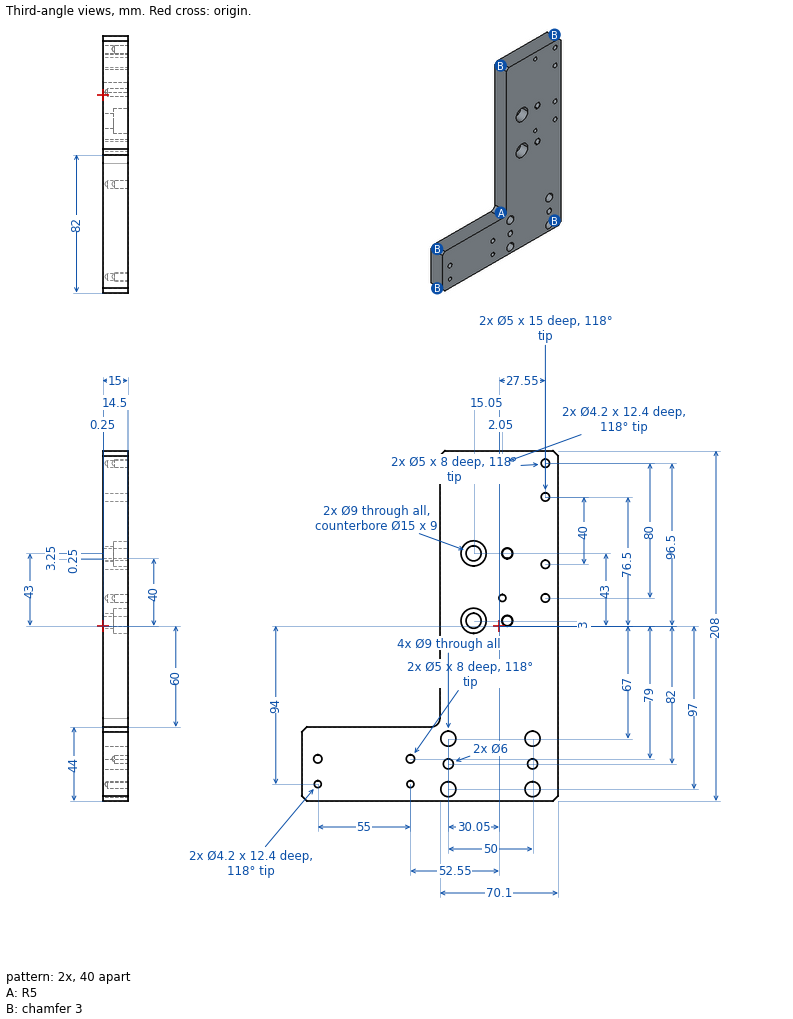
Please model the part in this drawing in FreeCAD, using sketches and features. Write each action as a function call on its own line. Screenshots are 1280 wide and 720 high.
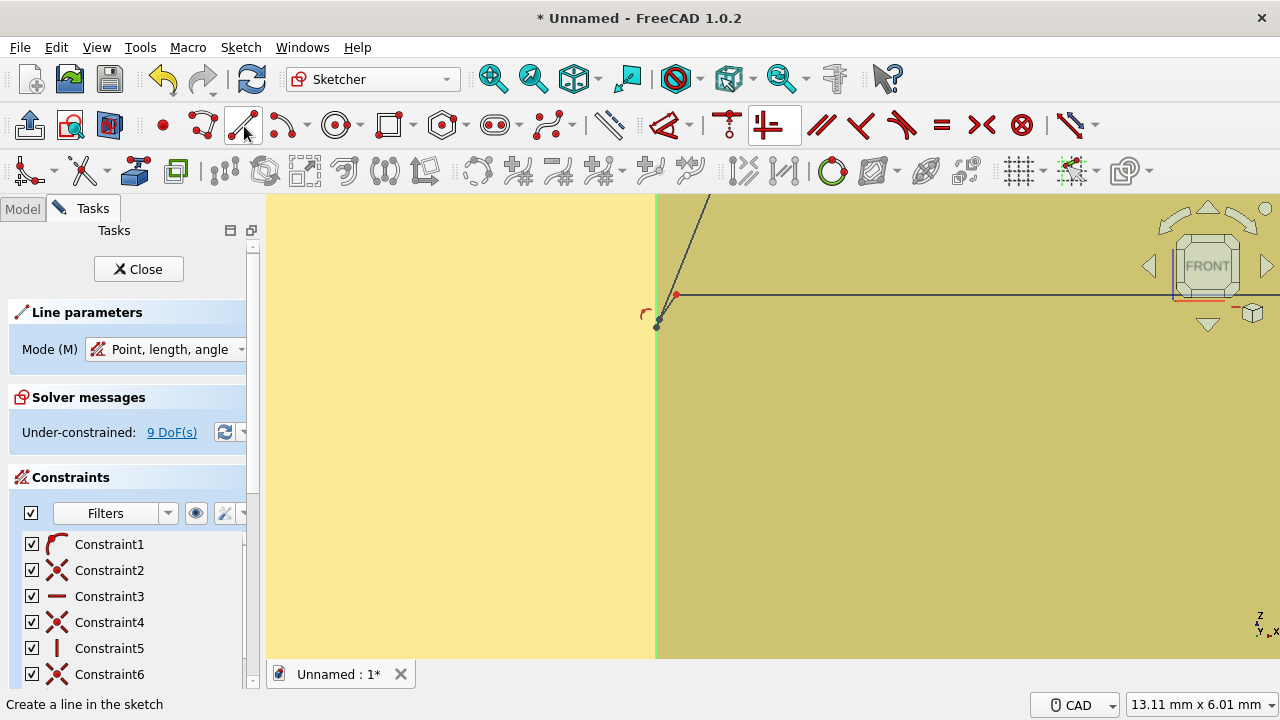
scroll(675, 297, down, 12)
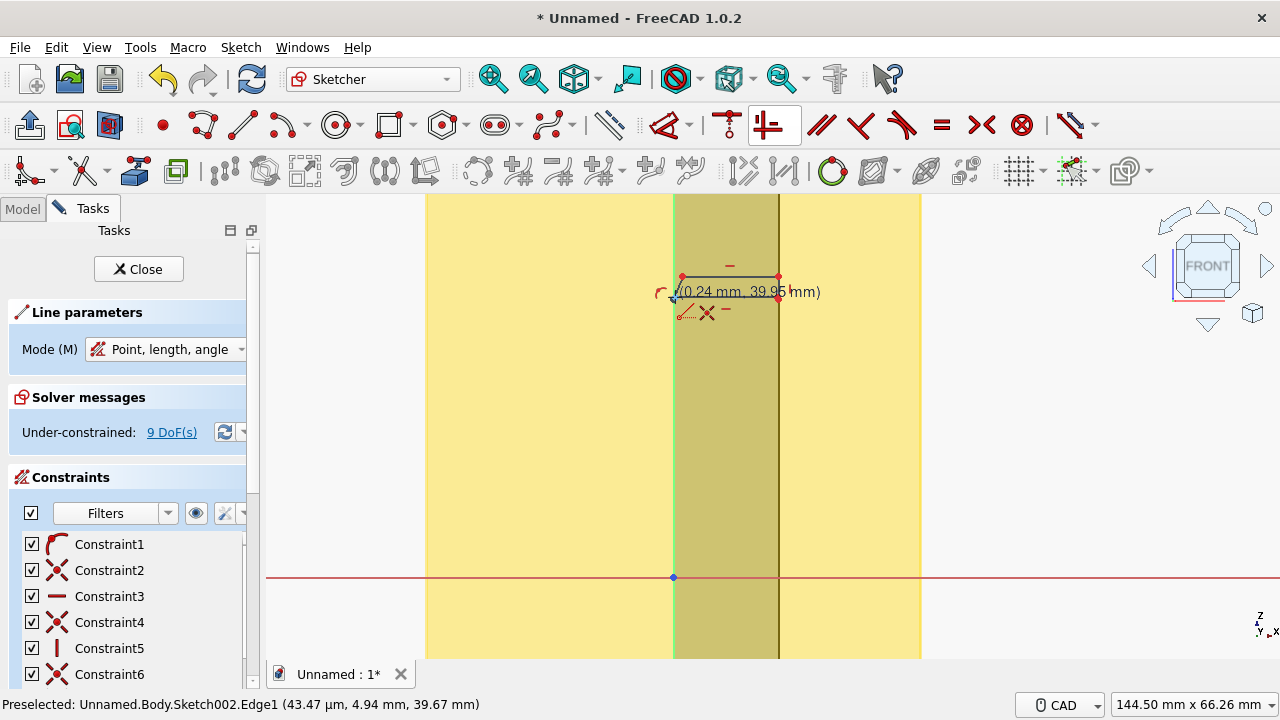
scroll(663, 276, up, 3)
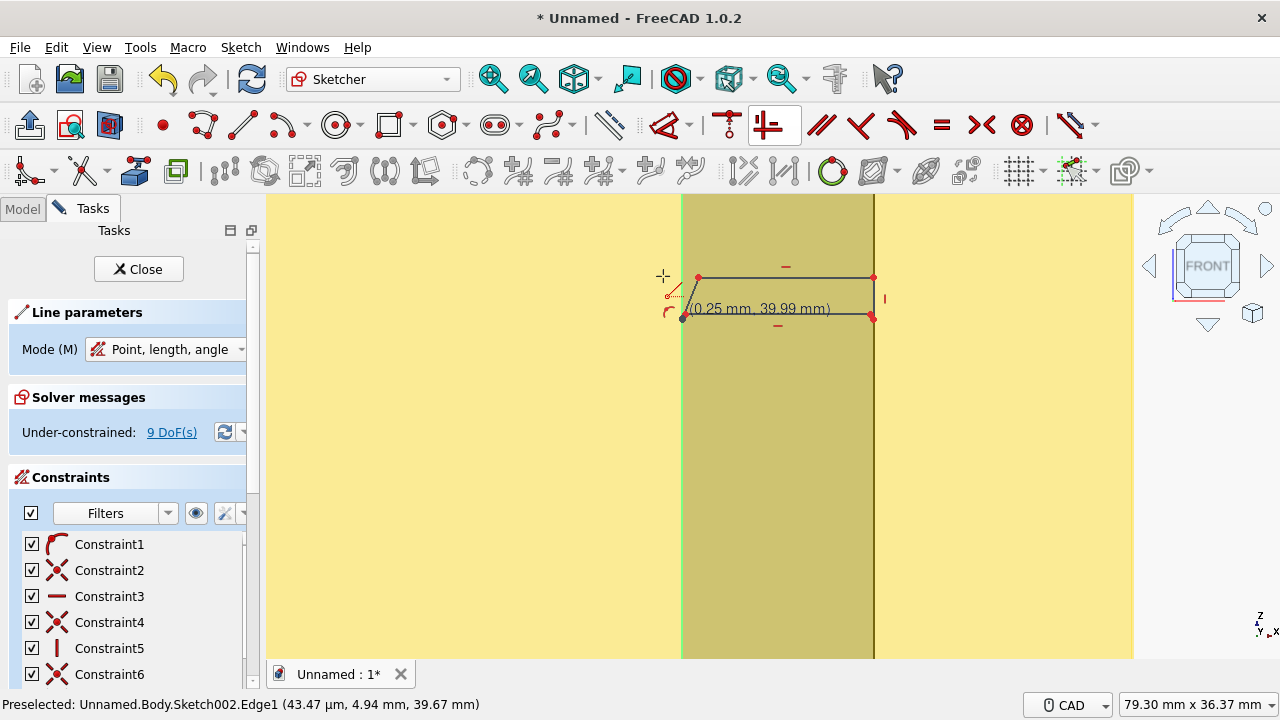
click(663, 276)
click(605, 276)
key(Escape)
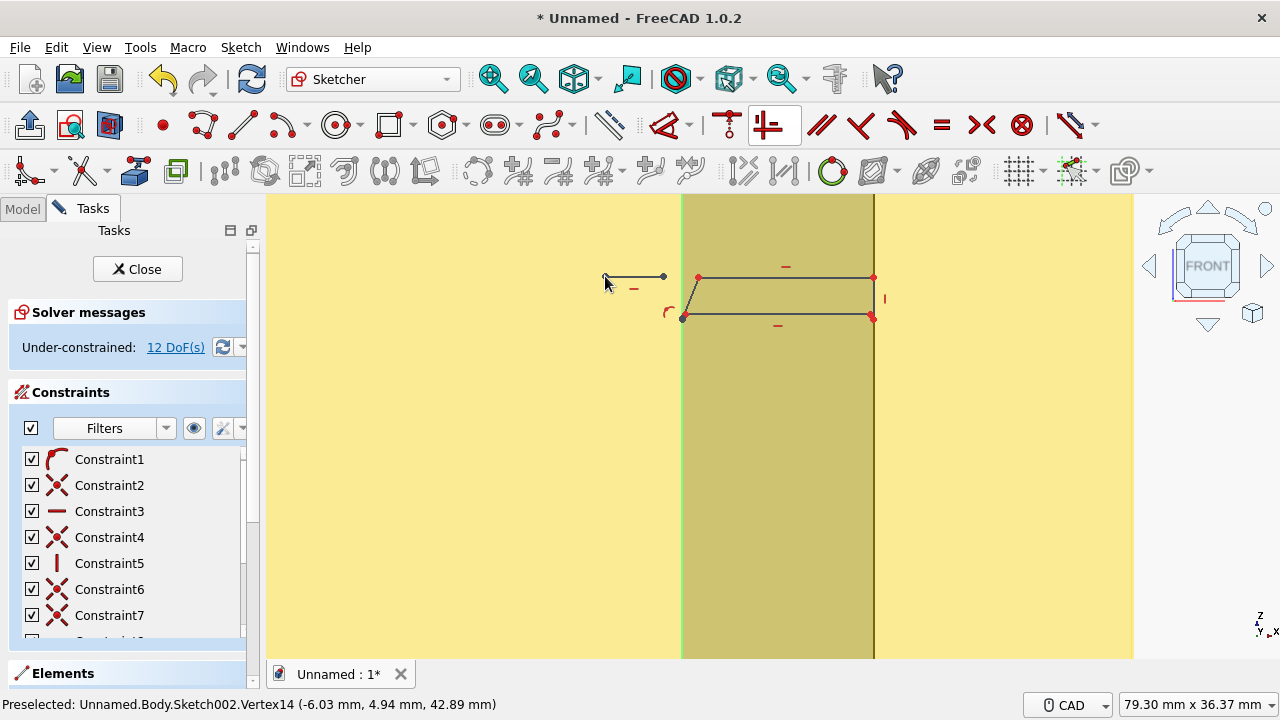
click(646, 277)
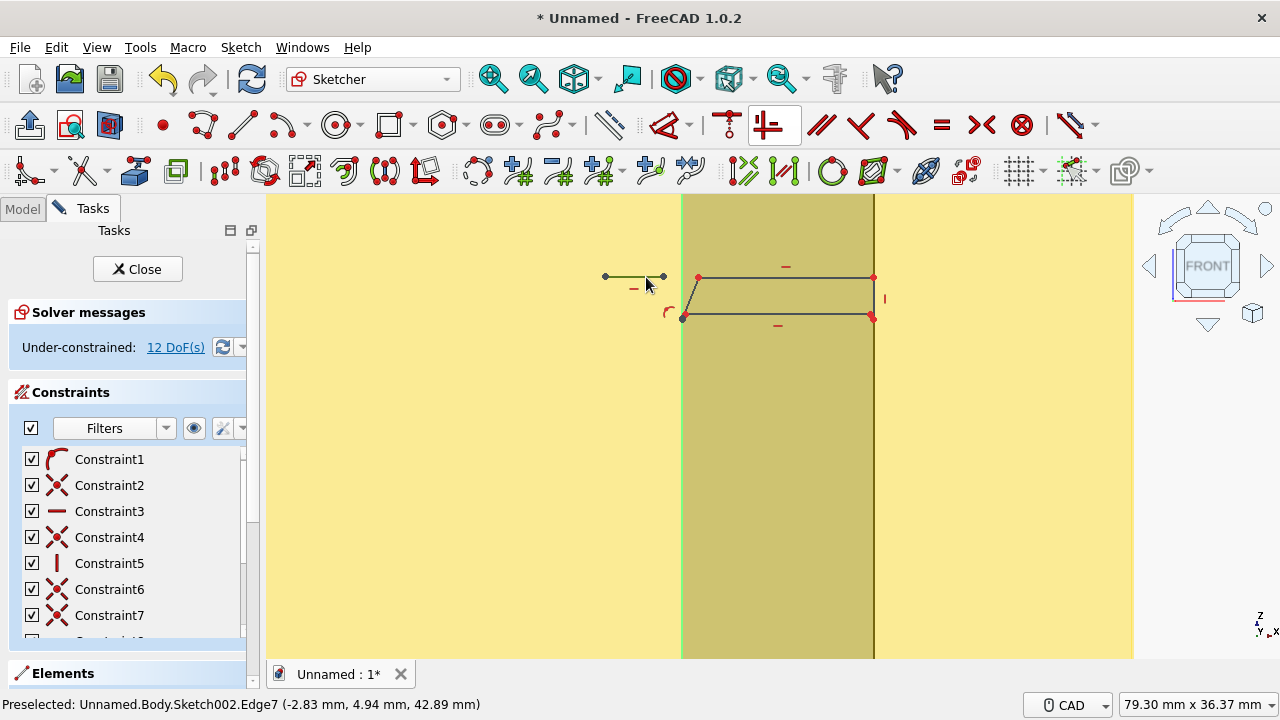
click(610, 126)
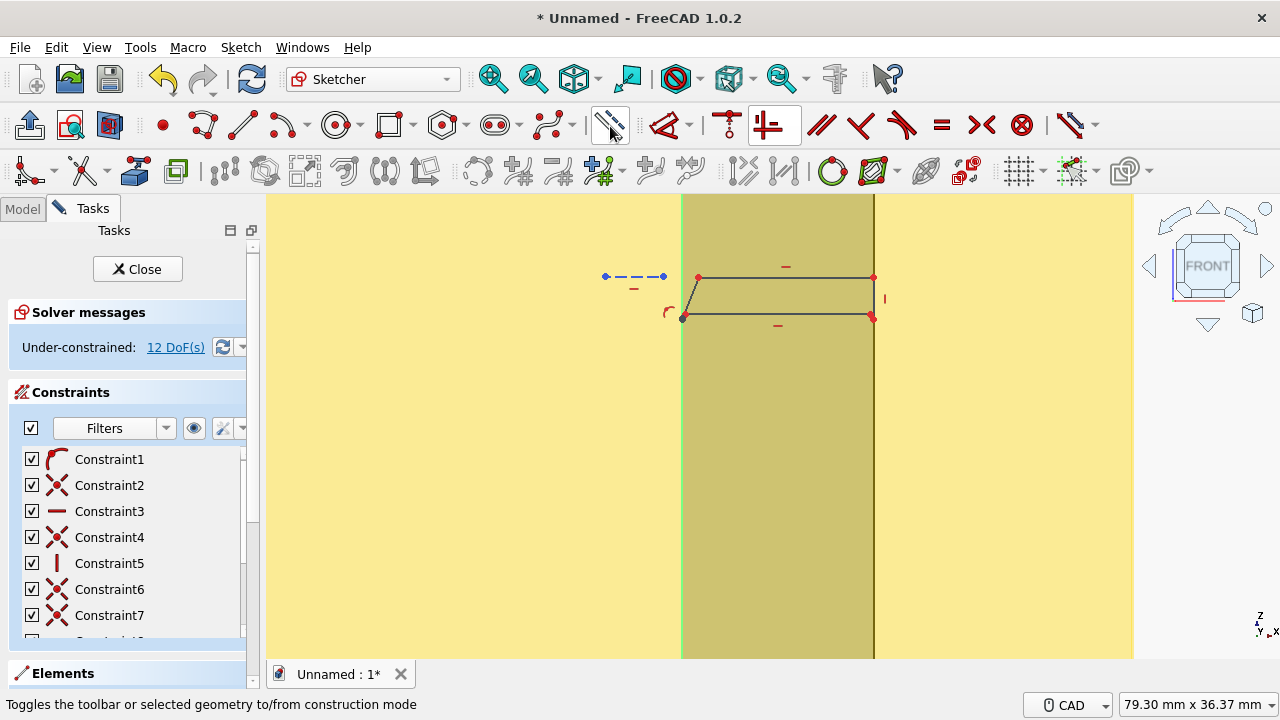
click(694, 290)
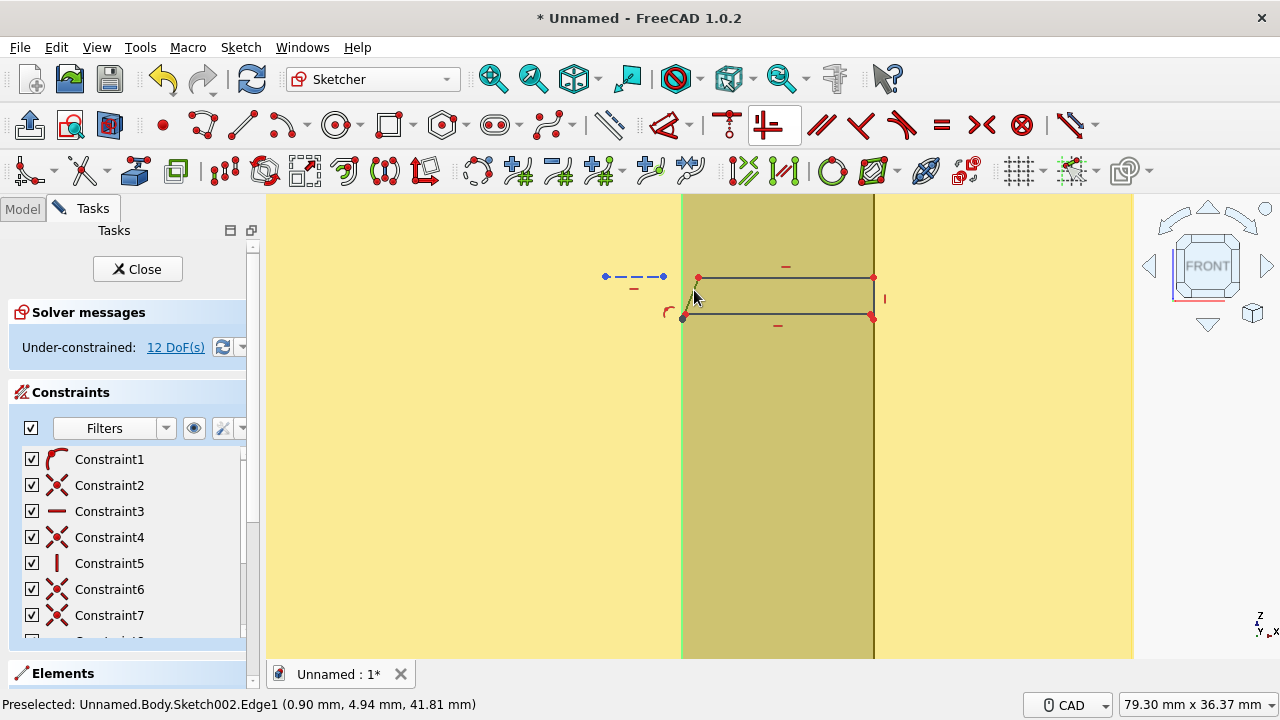
key(v)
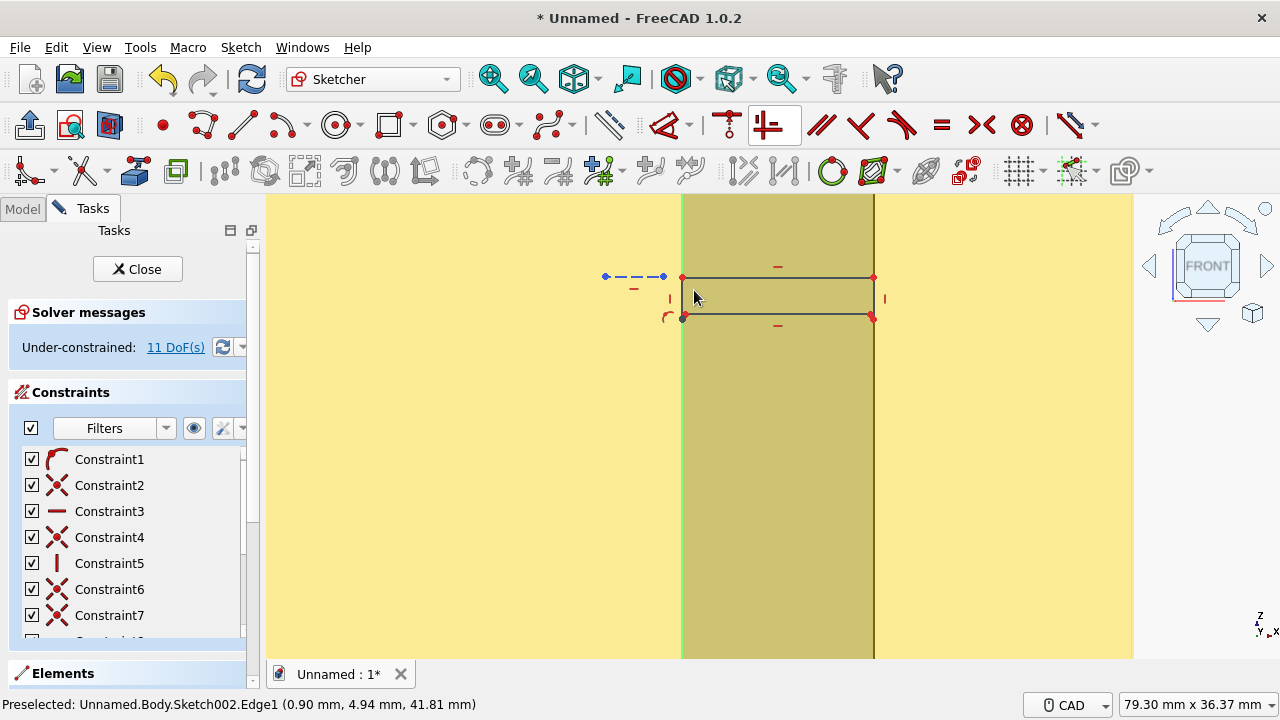
click(664, 126)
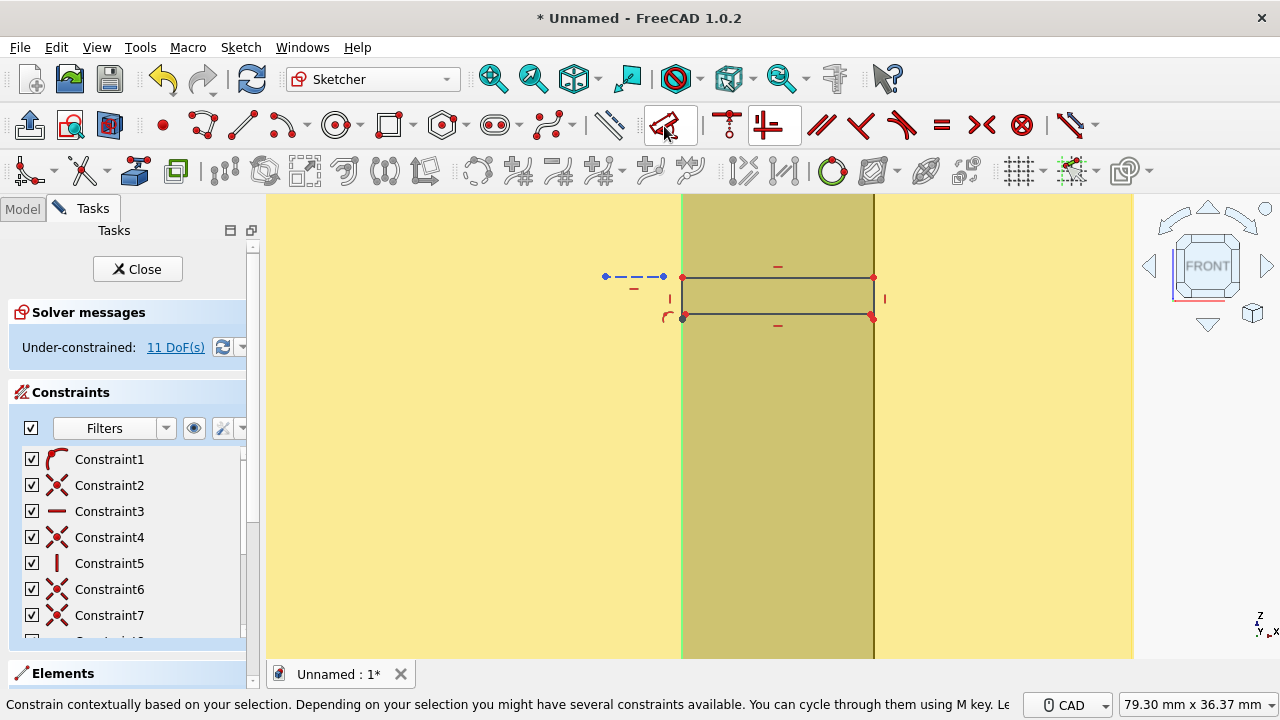
click(740, 278)
click(778, 244)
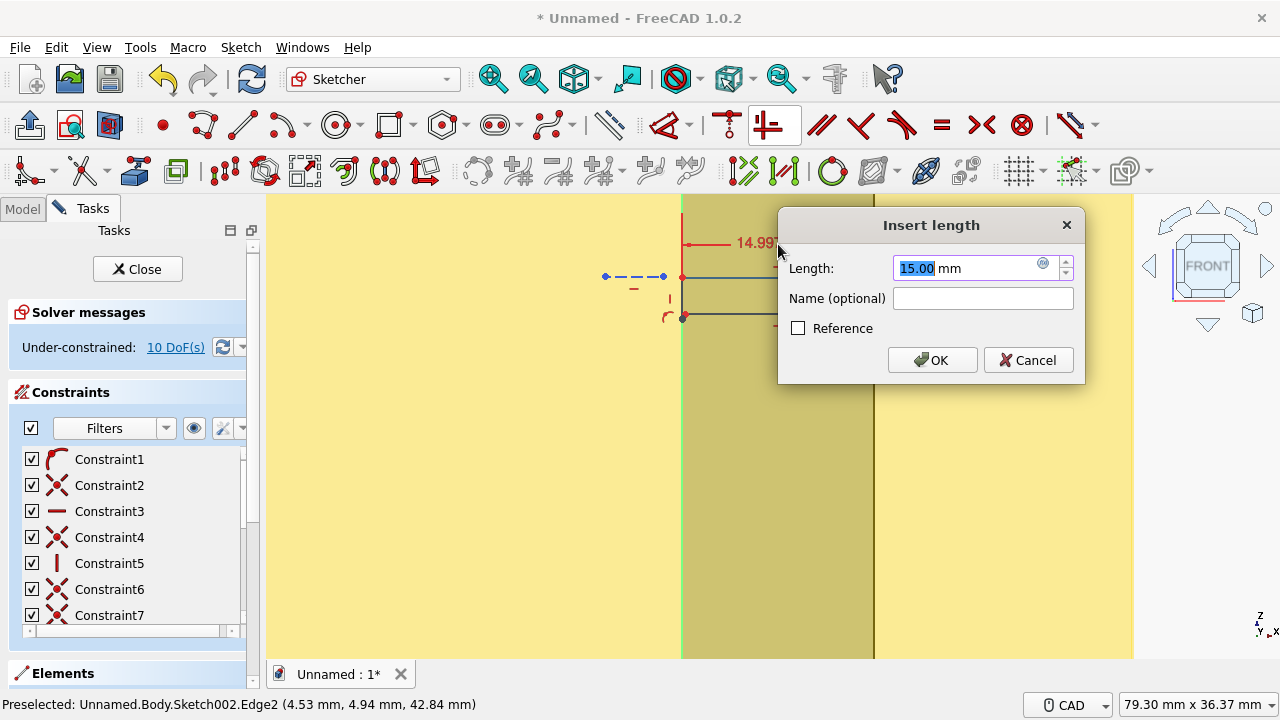
text(15)
key(Return)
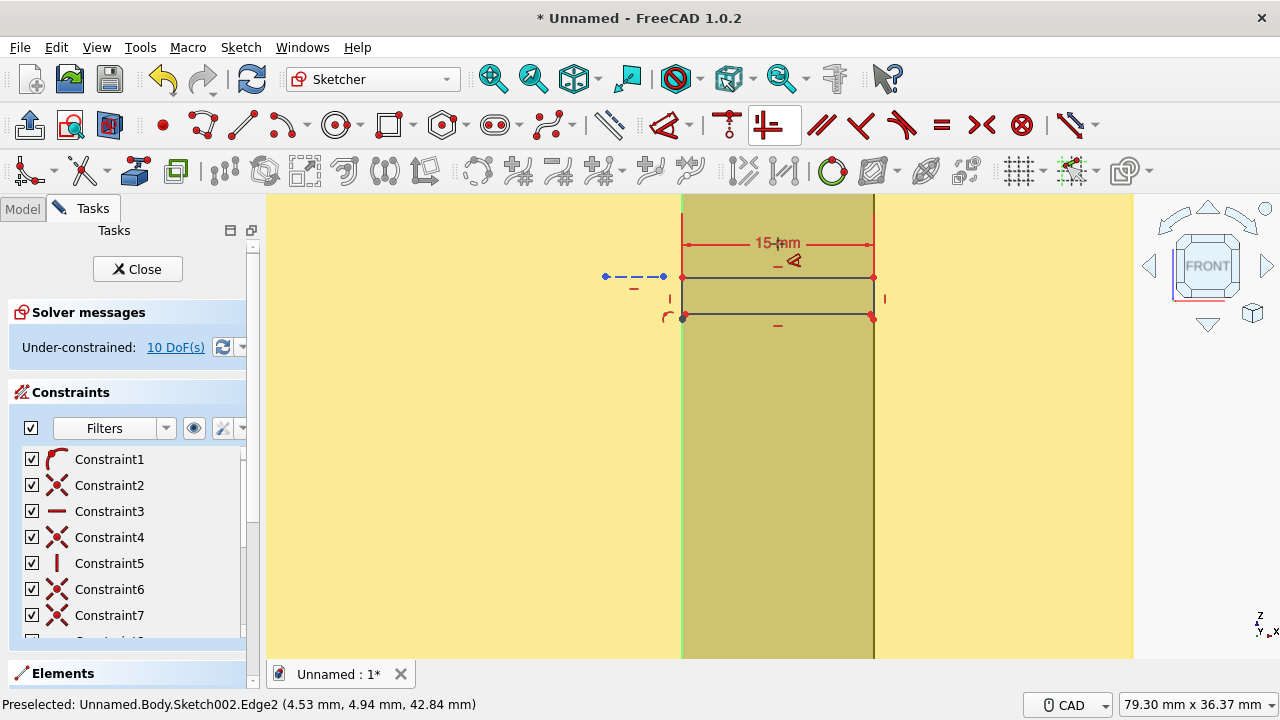
click(682, 278)
click(648, 454)